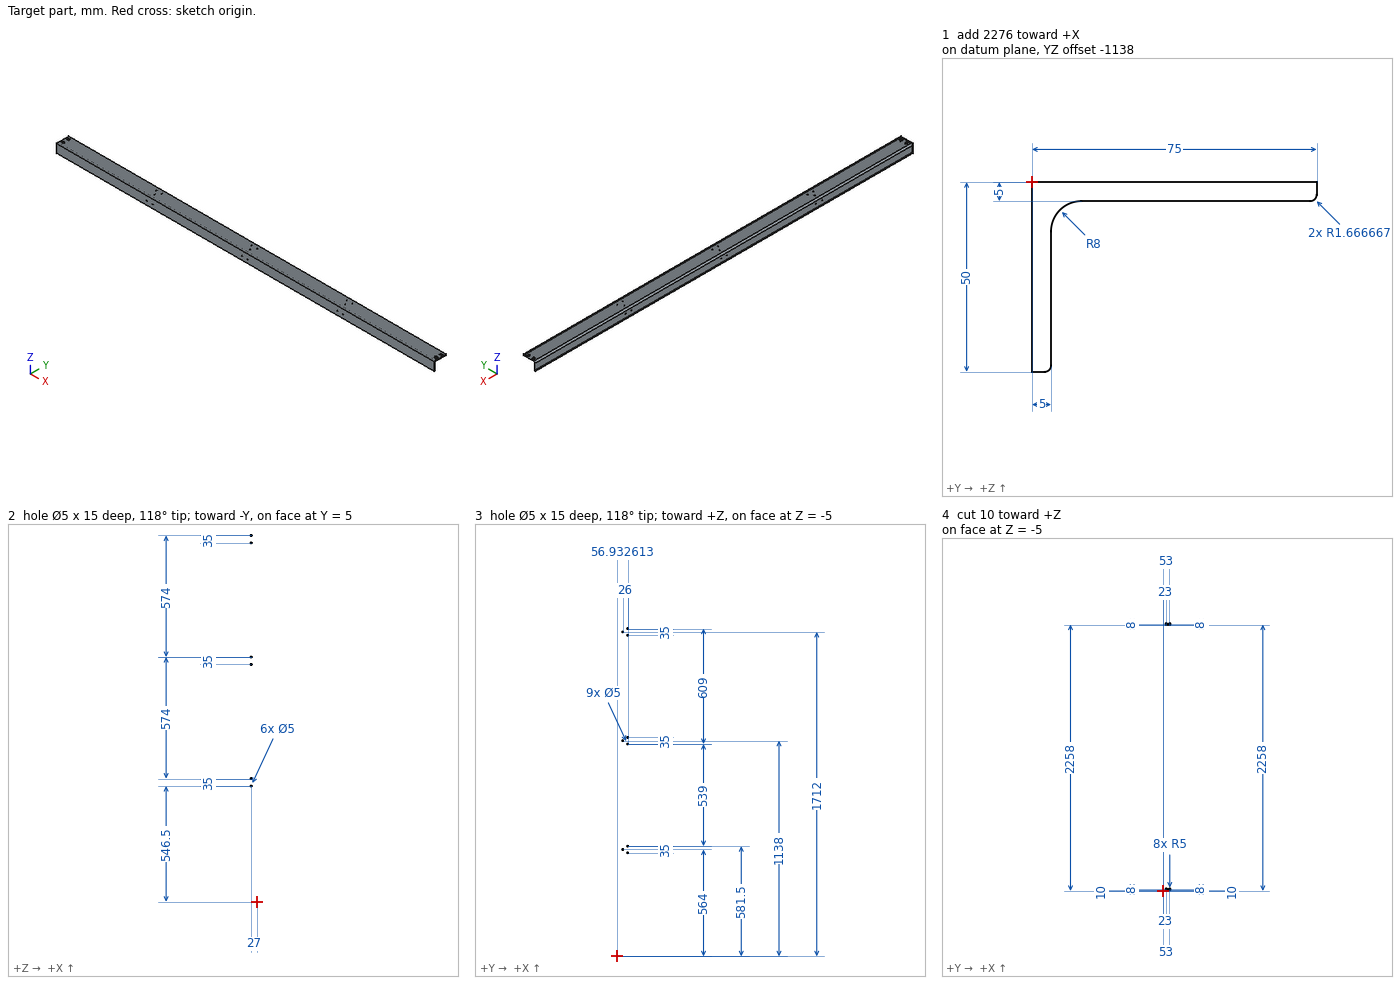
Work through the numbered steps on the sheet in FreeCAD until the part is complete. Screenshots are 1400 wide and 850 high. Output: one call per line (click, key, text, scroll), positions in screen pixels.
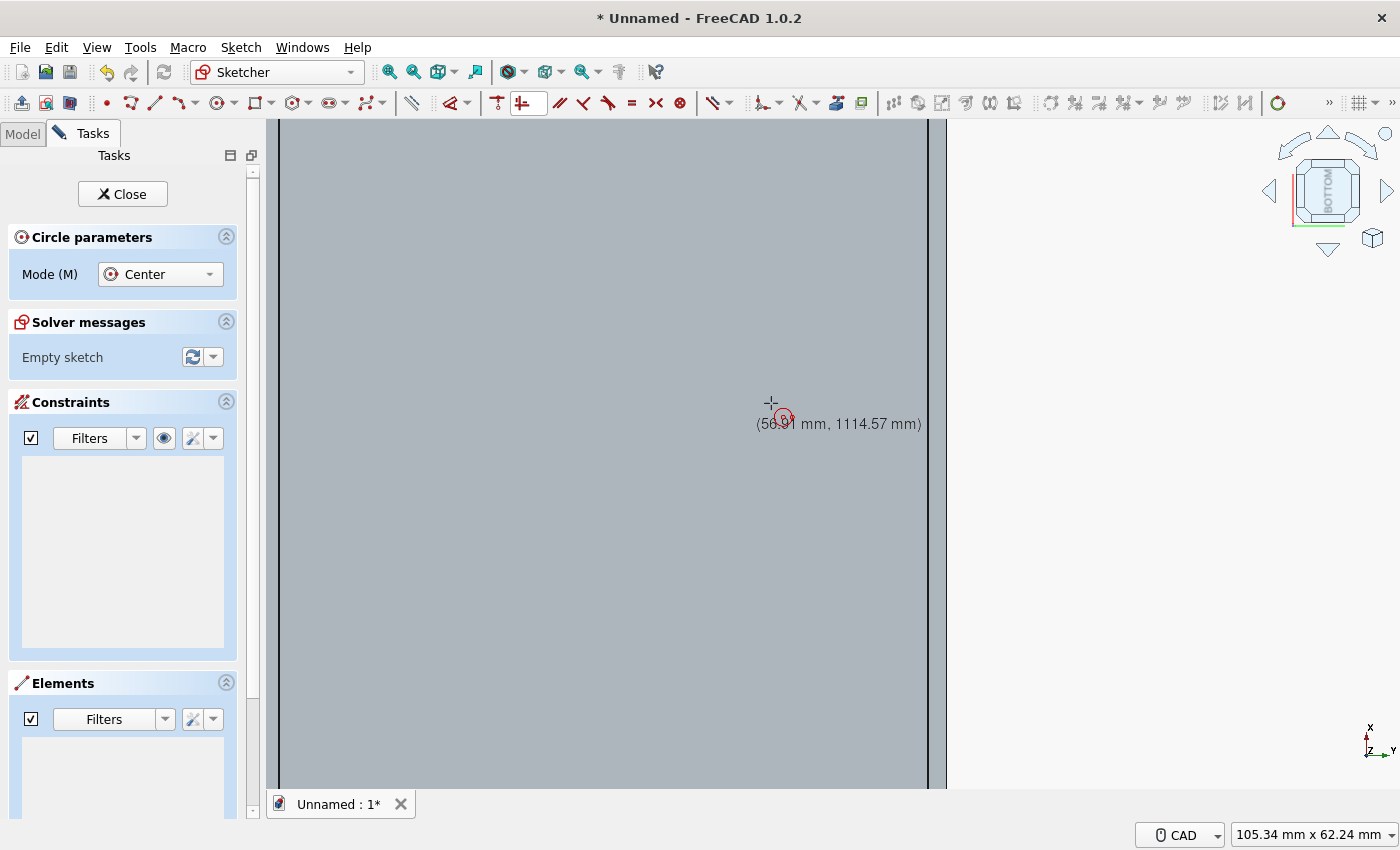
scroll(773, 380, down, 18)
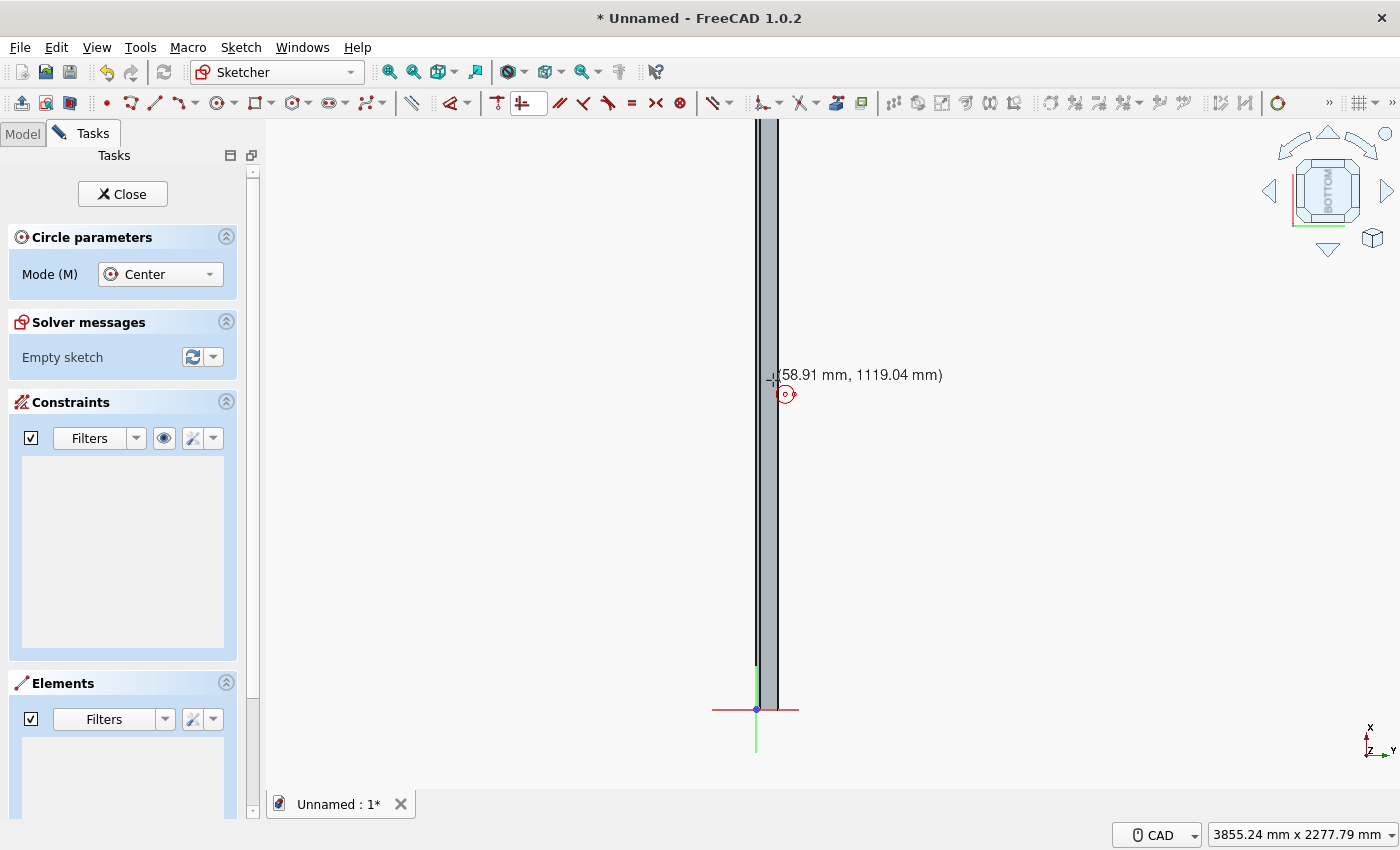
click(773, 380)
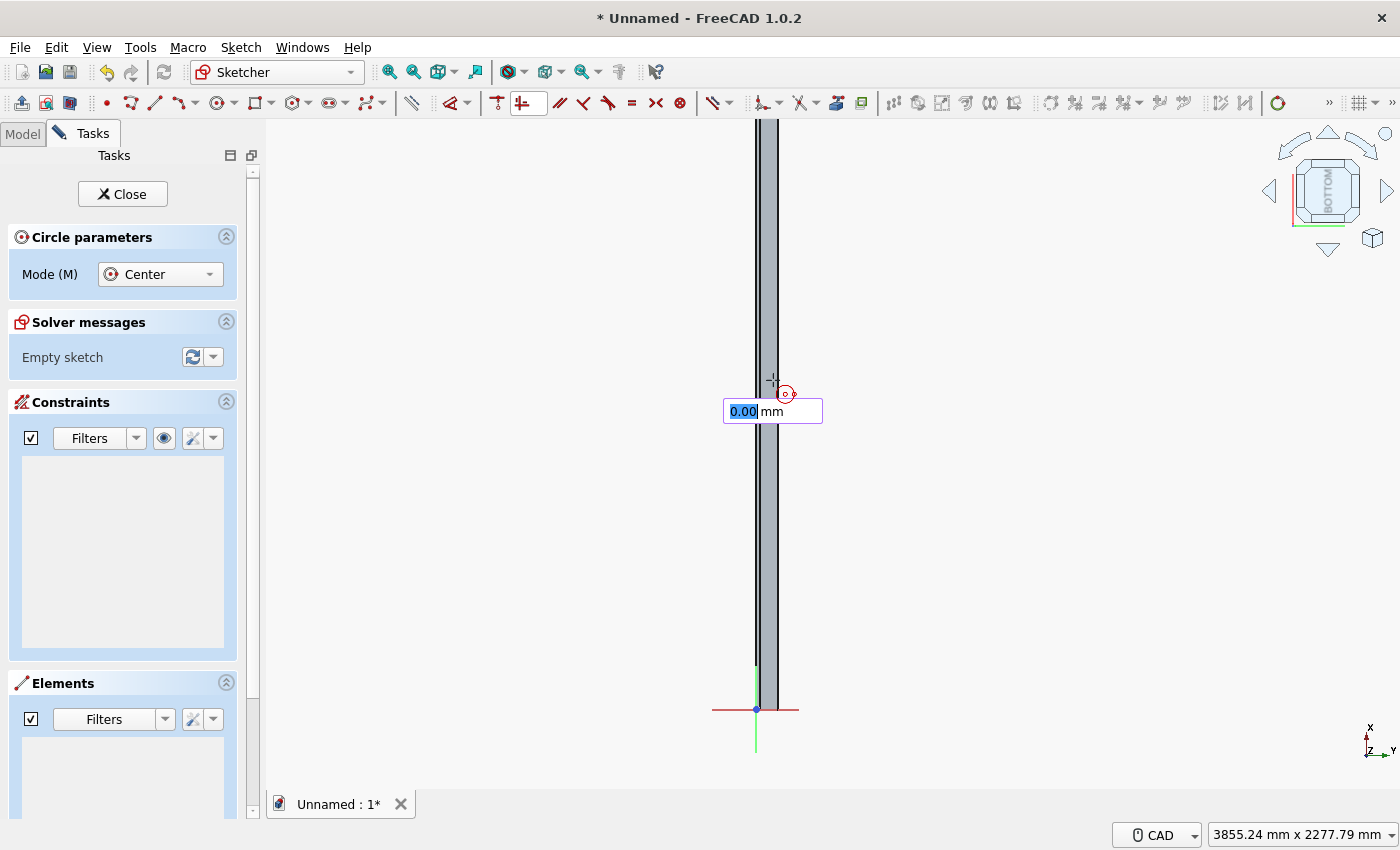
scroll(773, 379, up, 16)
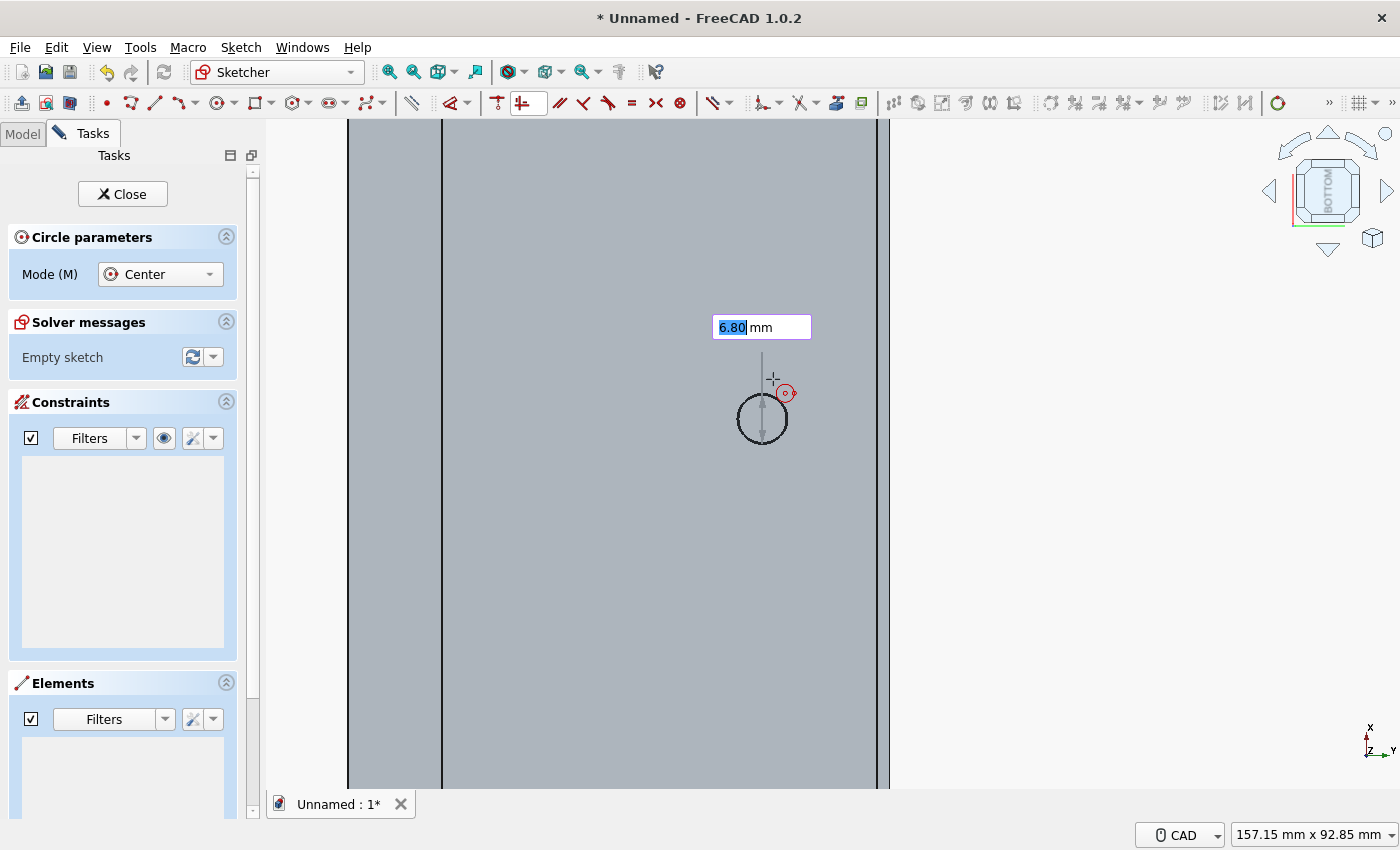
click(772, 381)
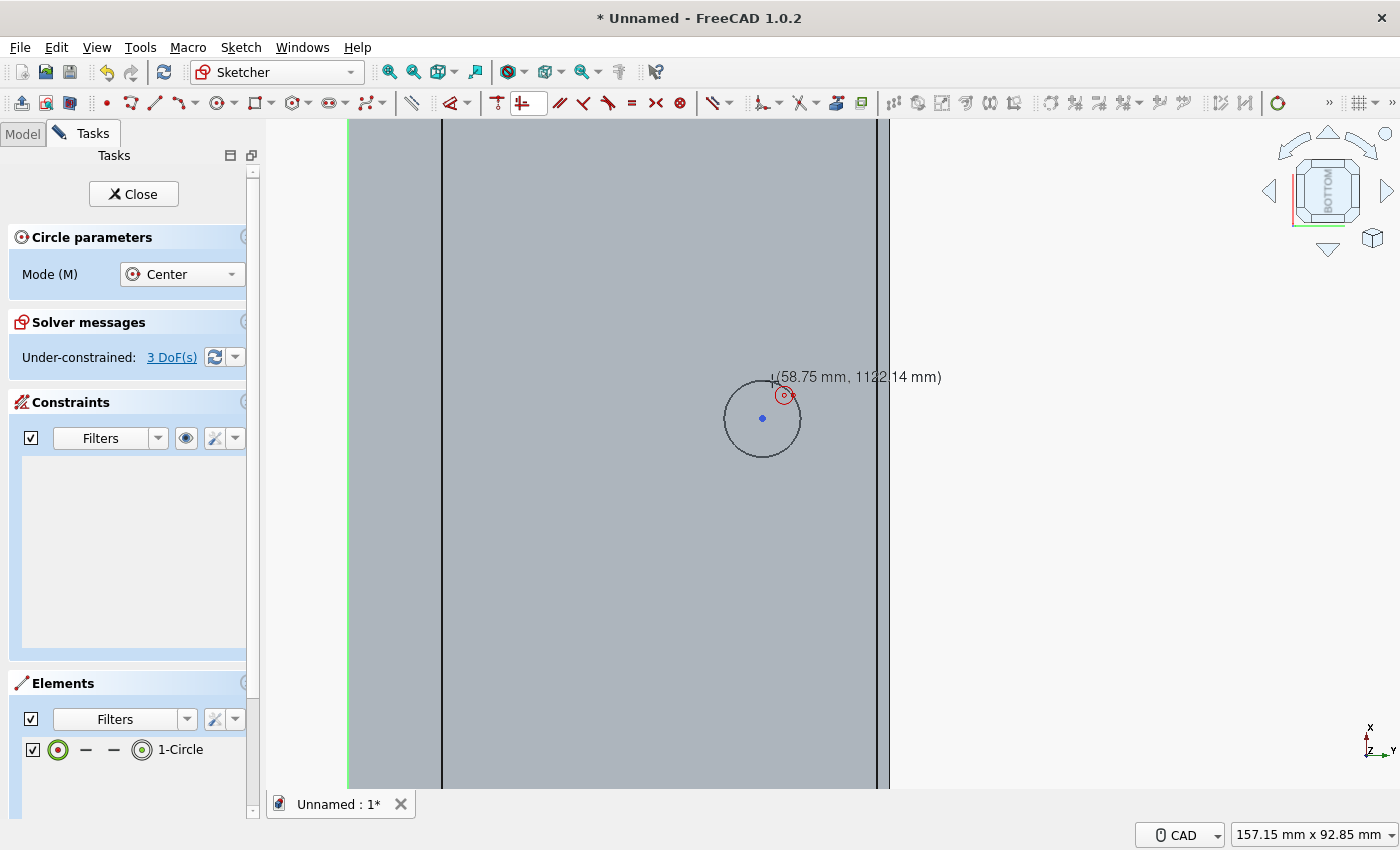
scroll(773, 379, down, 16)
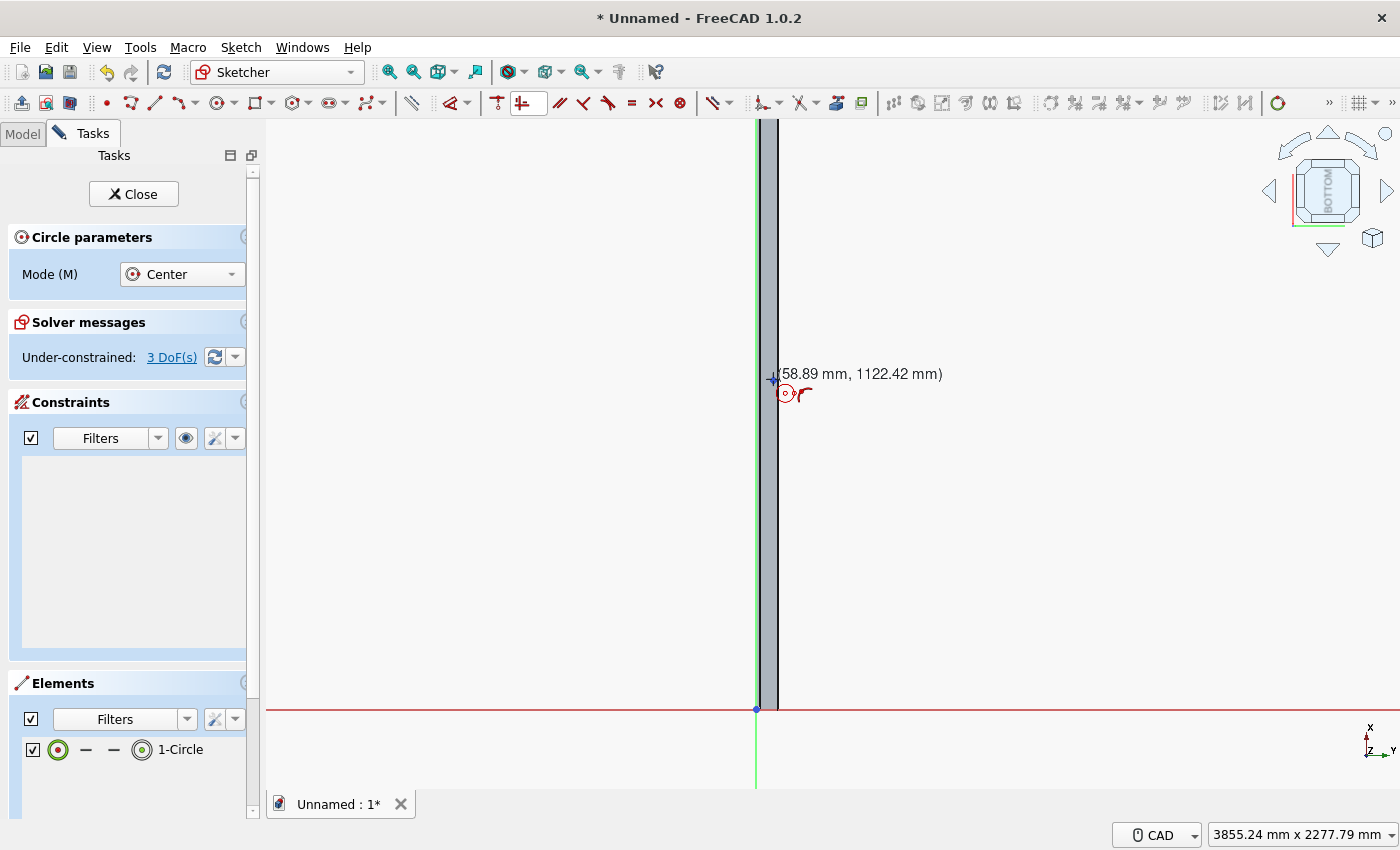
scroll(773, 201, up, 18)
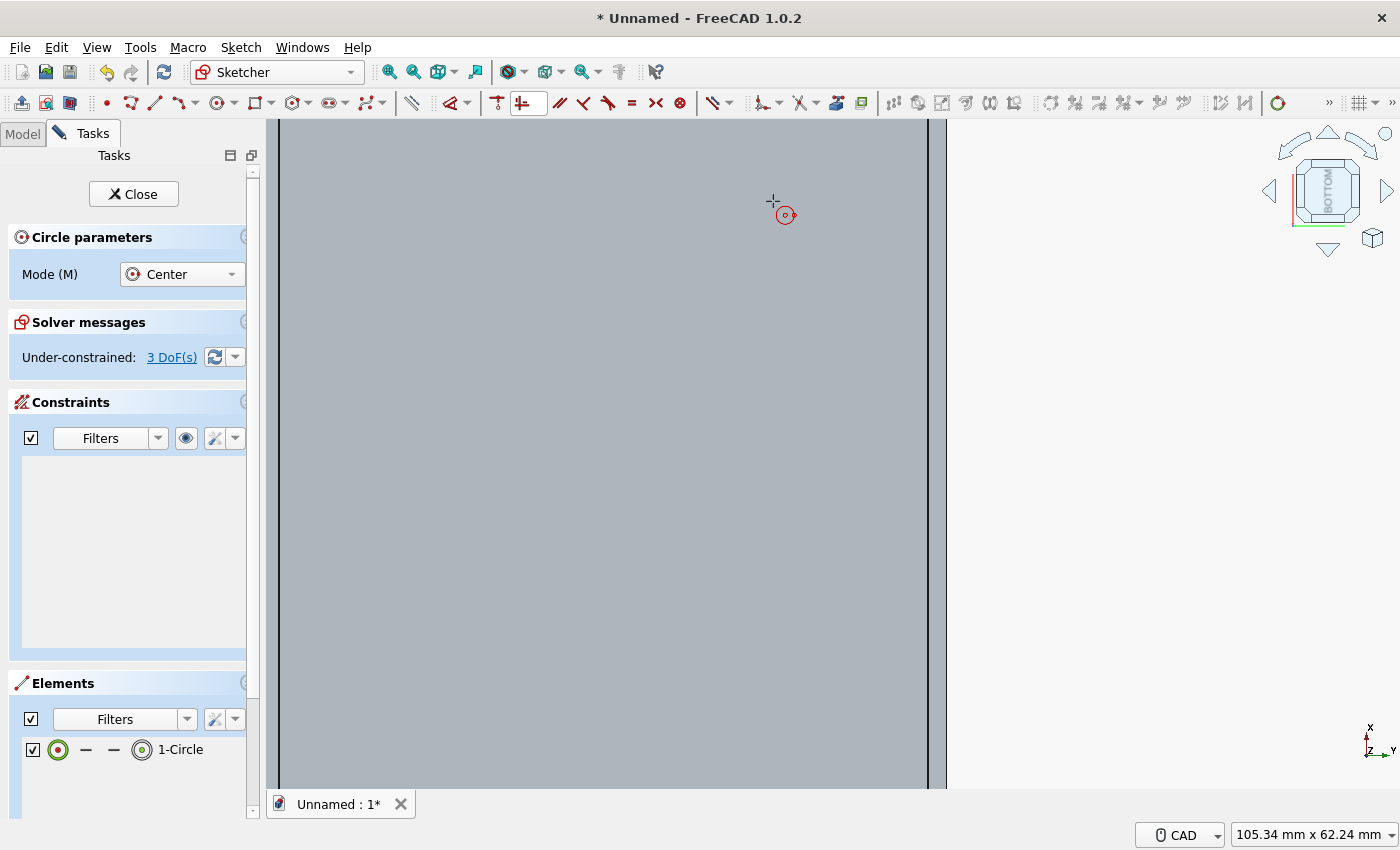
scroll(773, 200, down, 18)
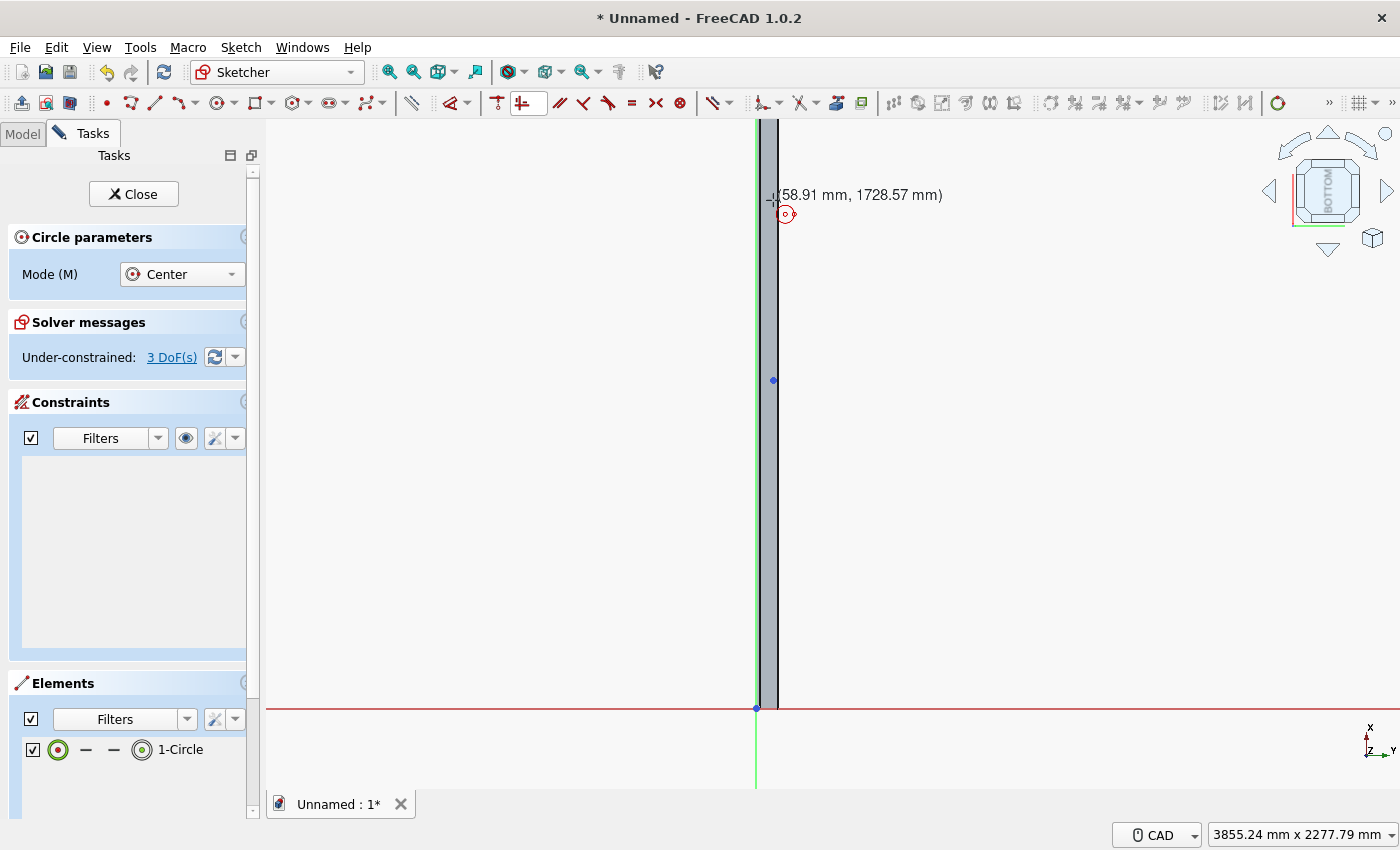
click(773, 200)